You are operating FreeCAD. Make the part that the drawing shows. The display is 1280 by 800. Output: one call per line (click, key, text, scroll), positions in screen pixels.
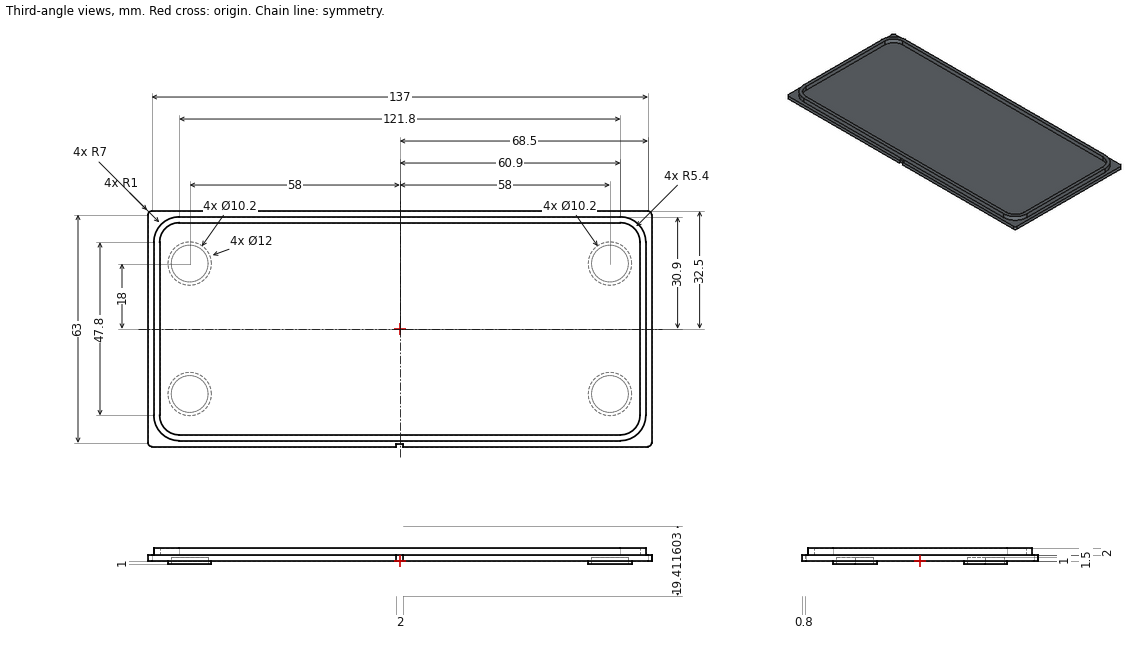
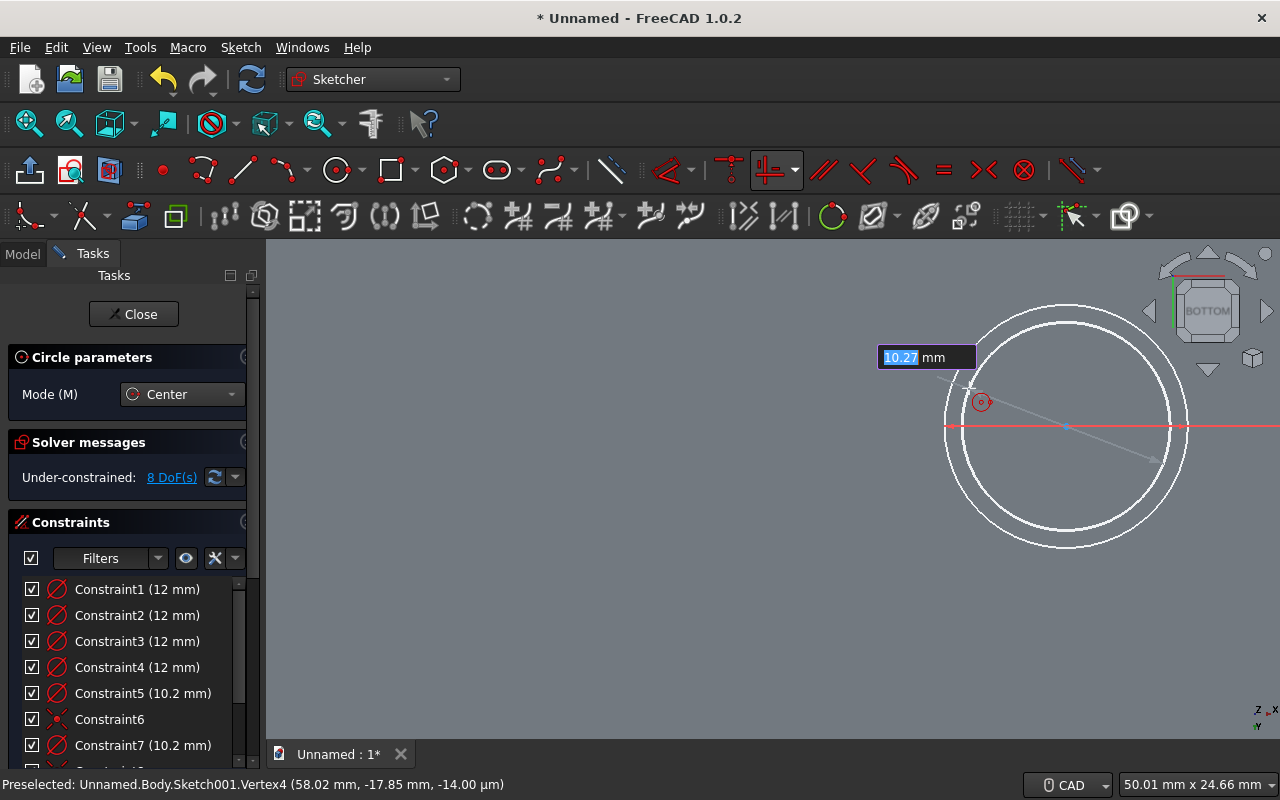
text(10.2)
key(Return)
key(Escape)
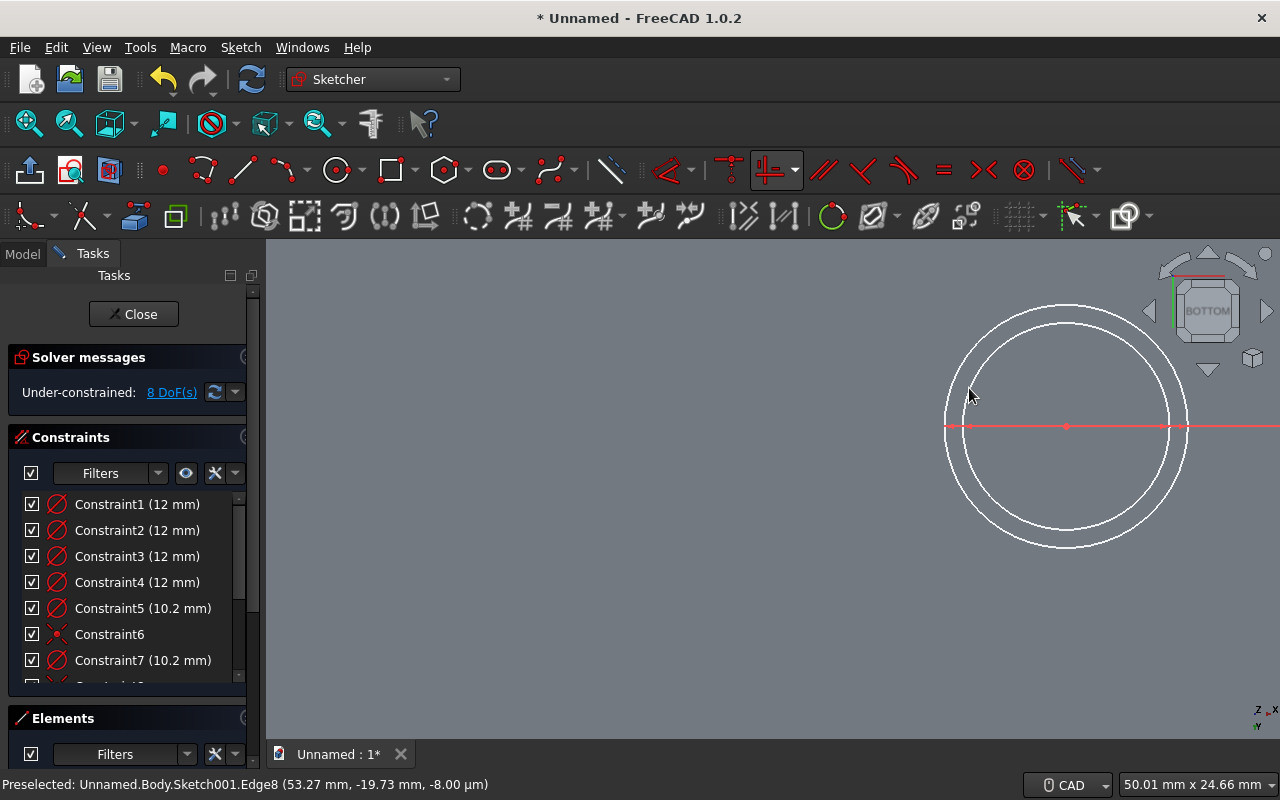
scroll(971, 391, down, 7)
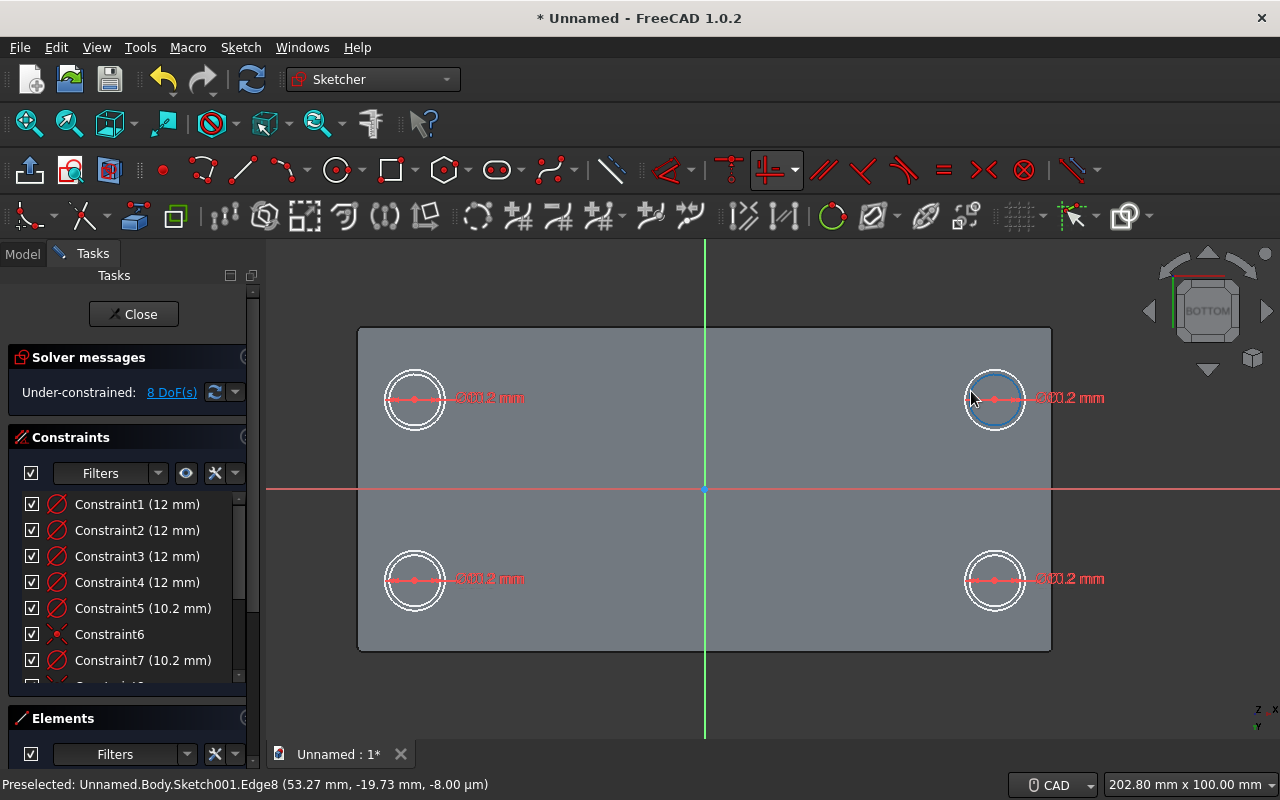
click(415, 581)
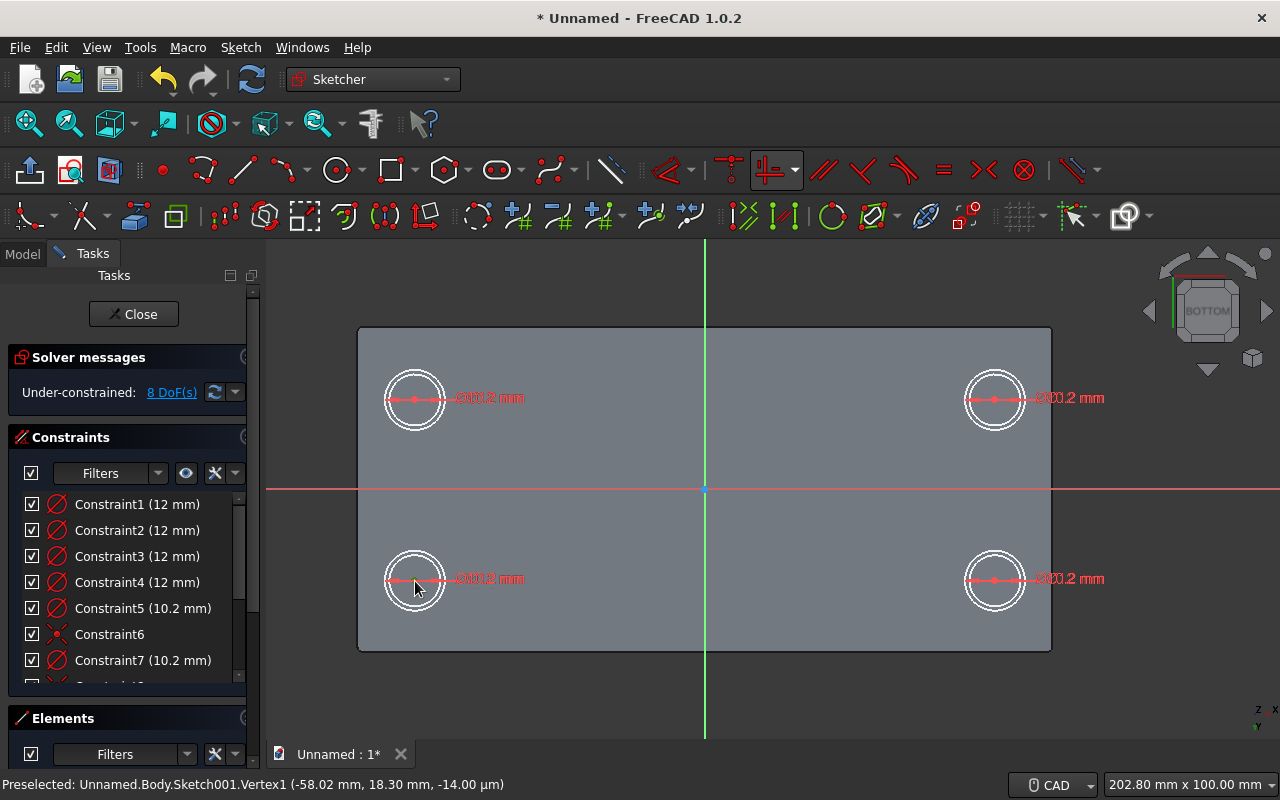
click(995, 581)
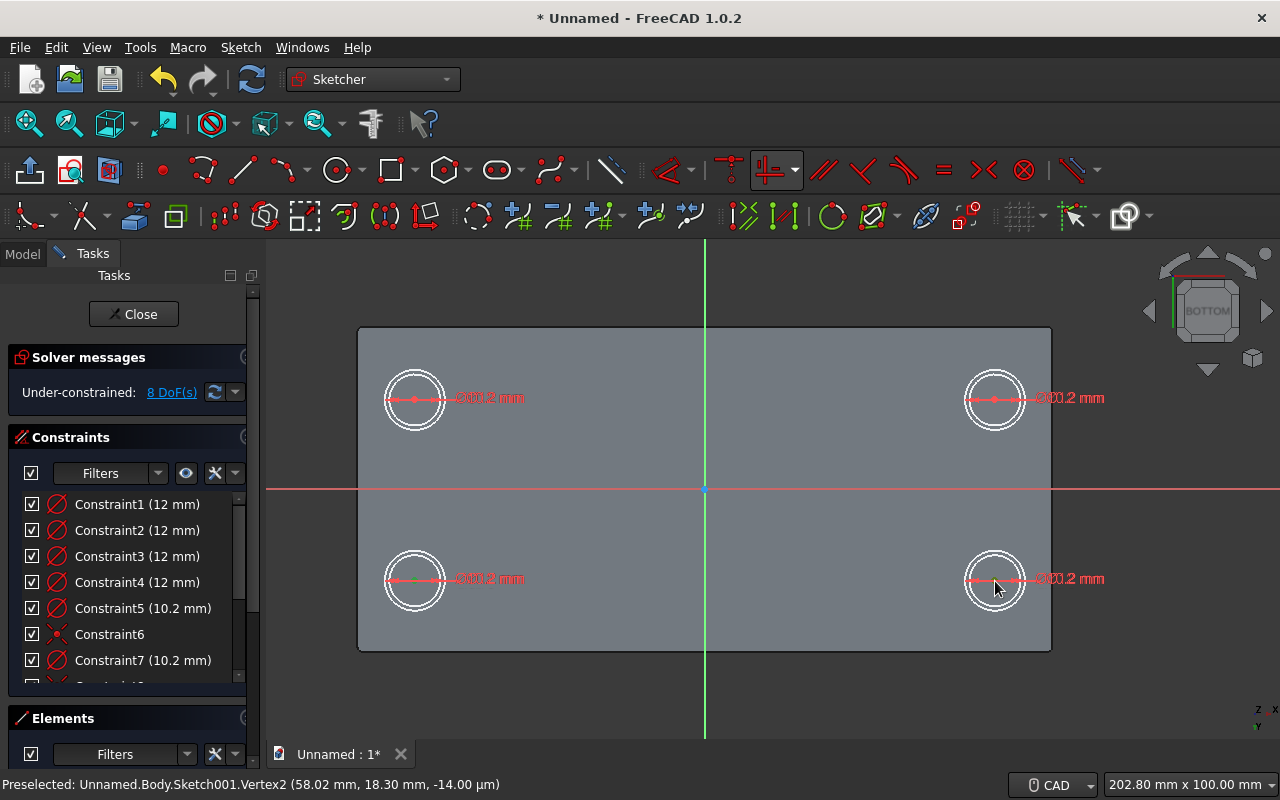
click(705, 679)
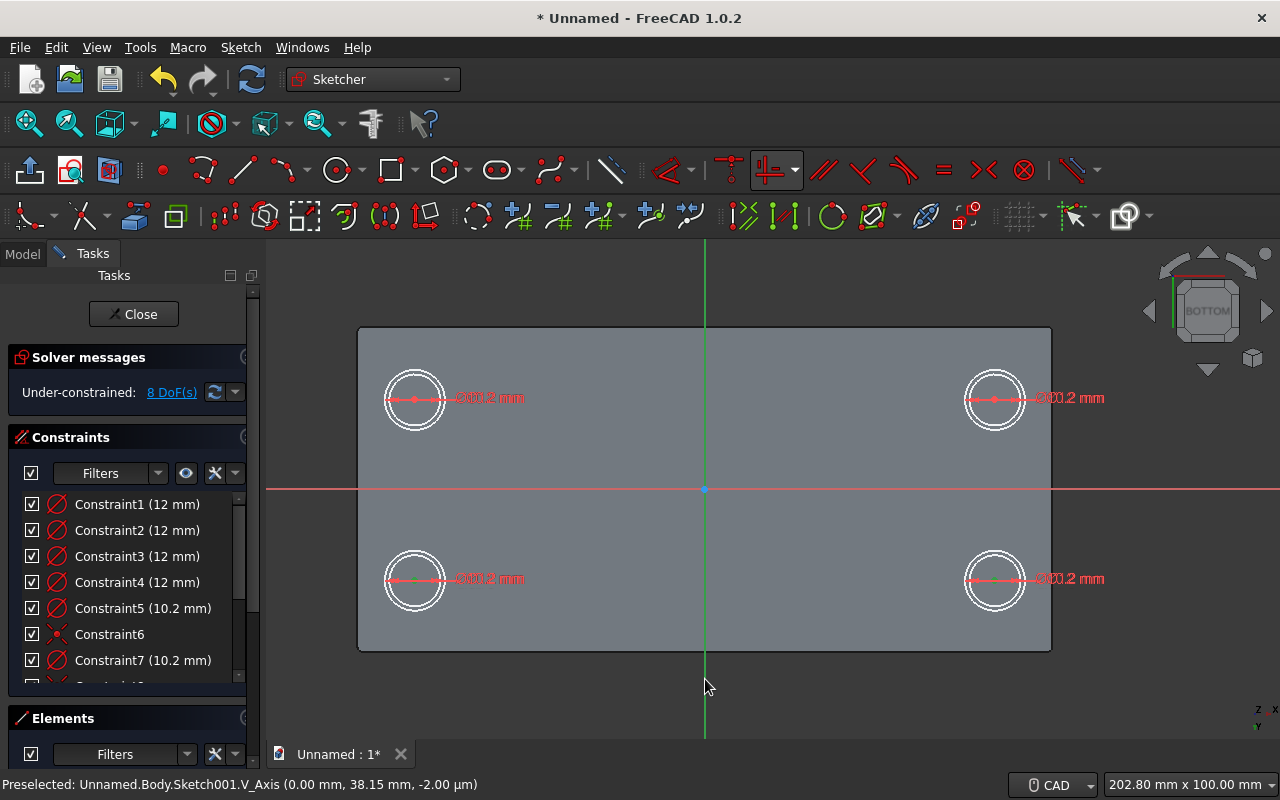
click(984, 170)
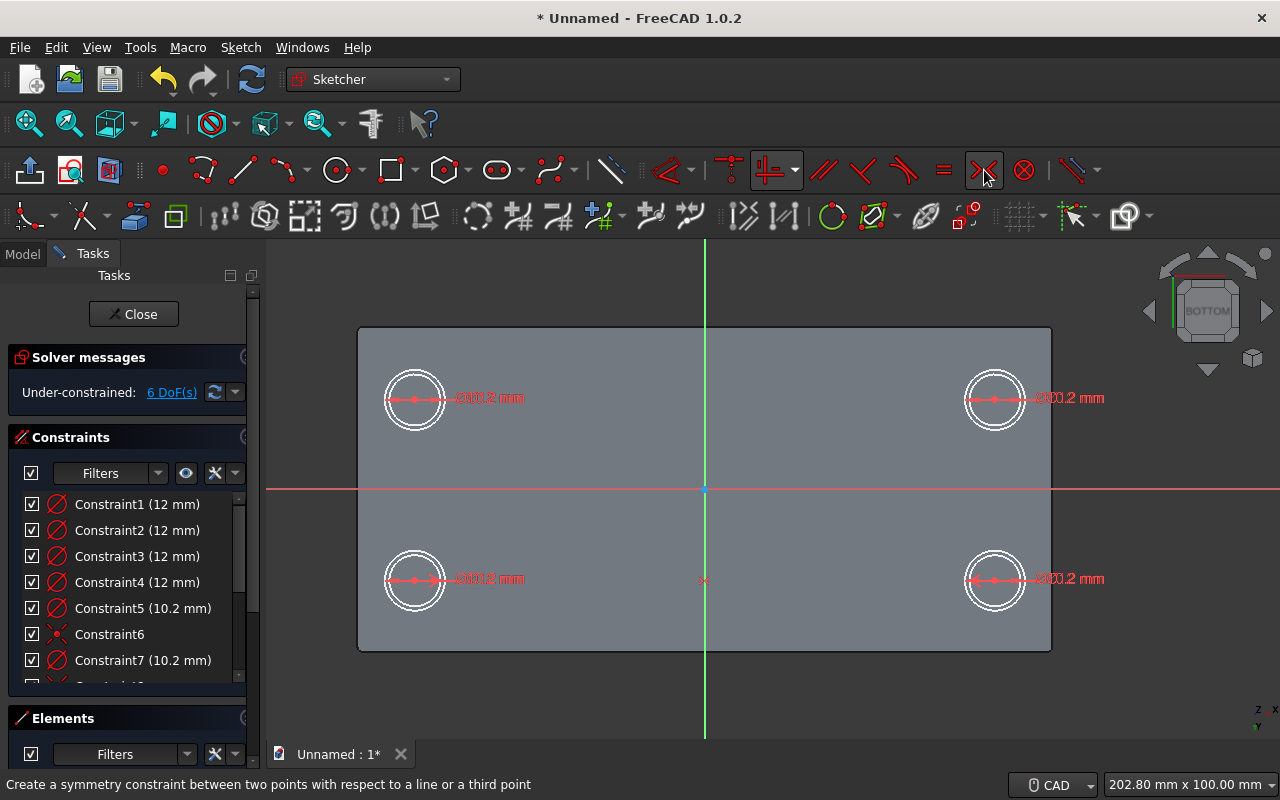
click(415, 581)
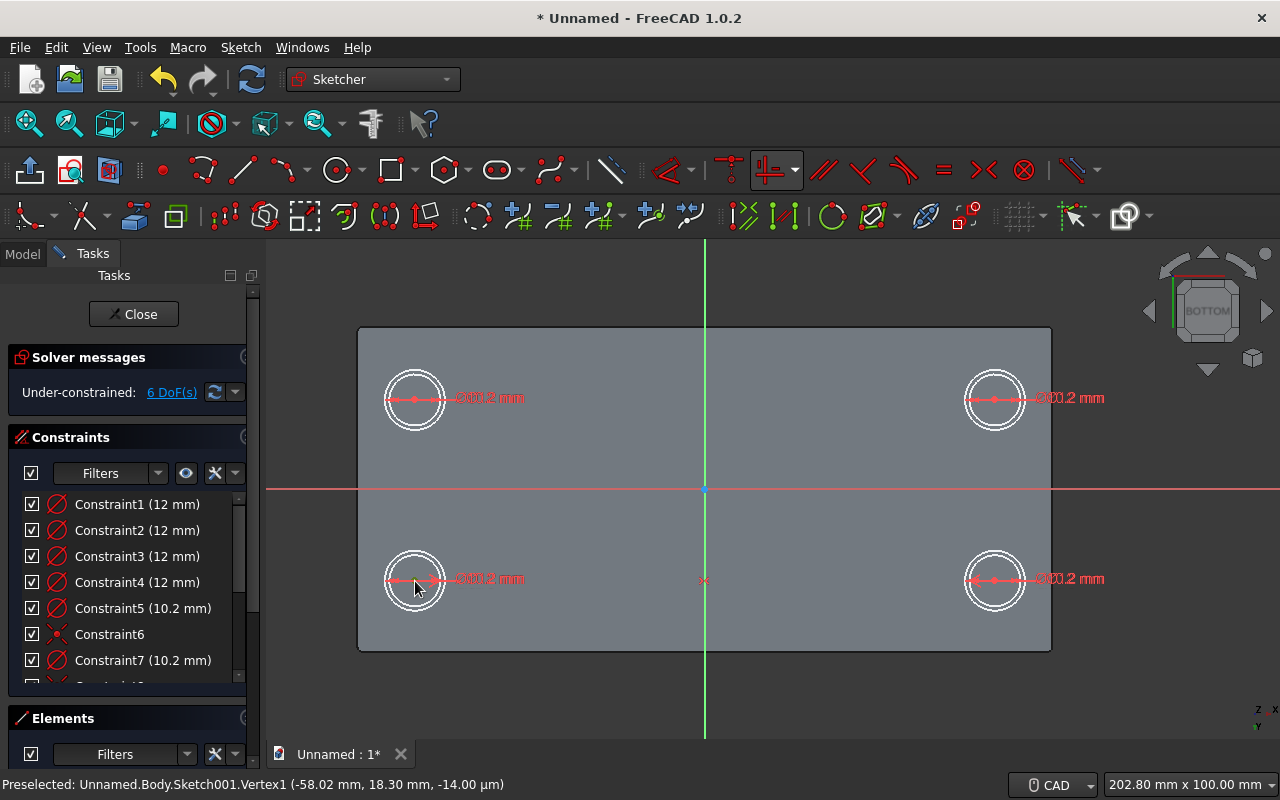
click(415, 400)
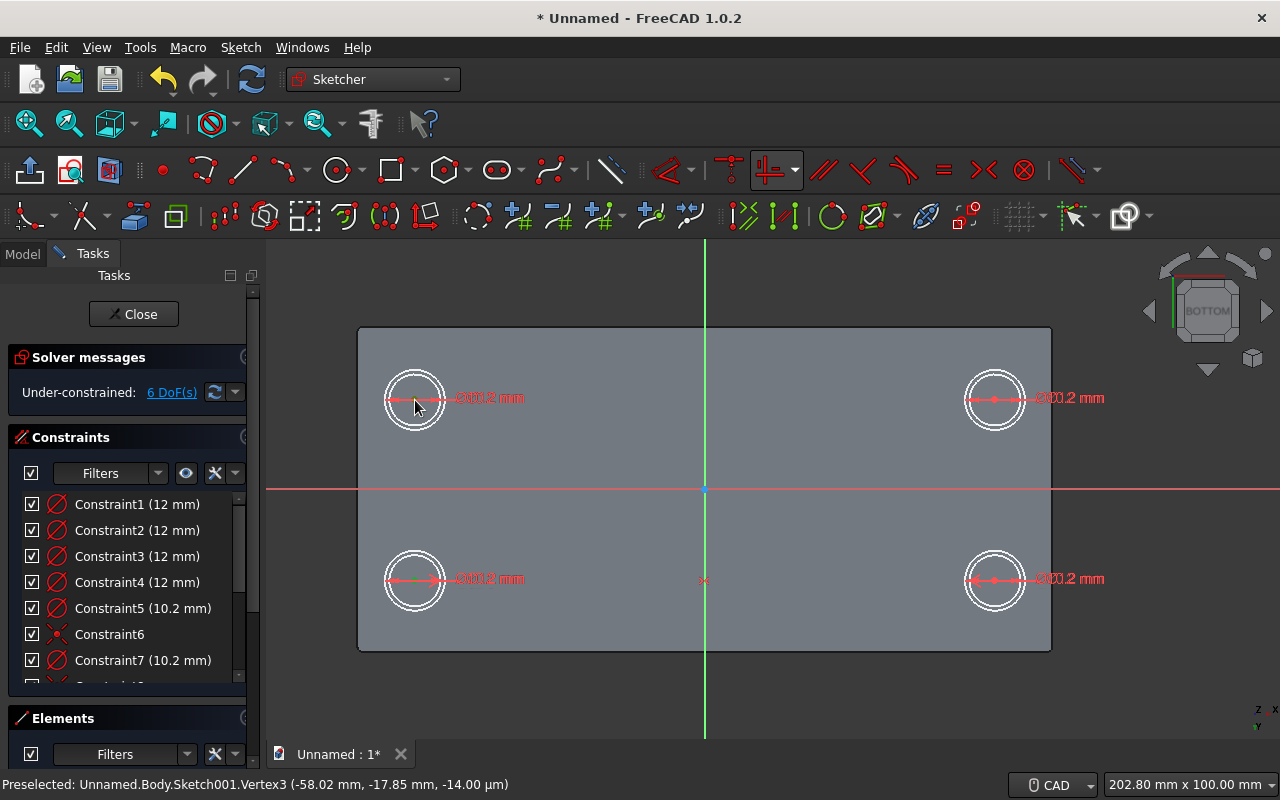
click(353, 489)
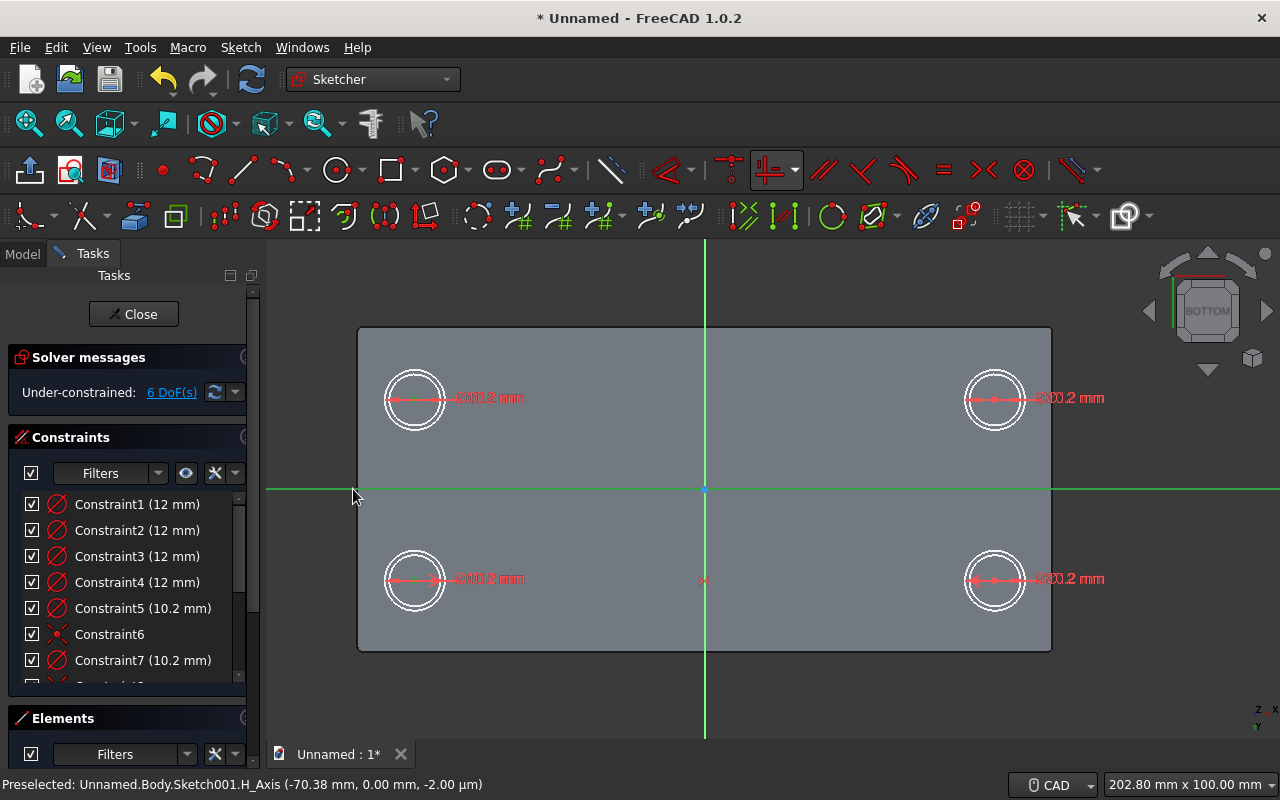
click(984, 170)